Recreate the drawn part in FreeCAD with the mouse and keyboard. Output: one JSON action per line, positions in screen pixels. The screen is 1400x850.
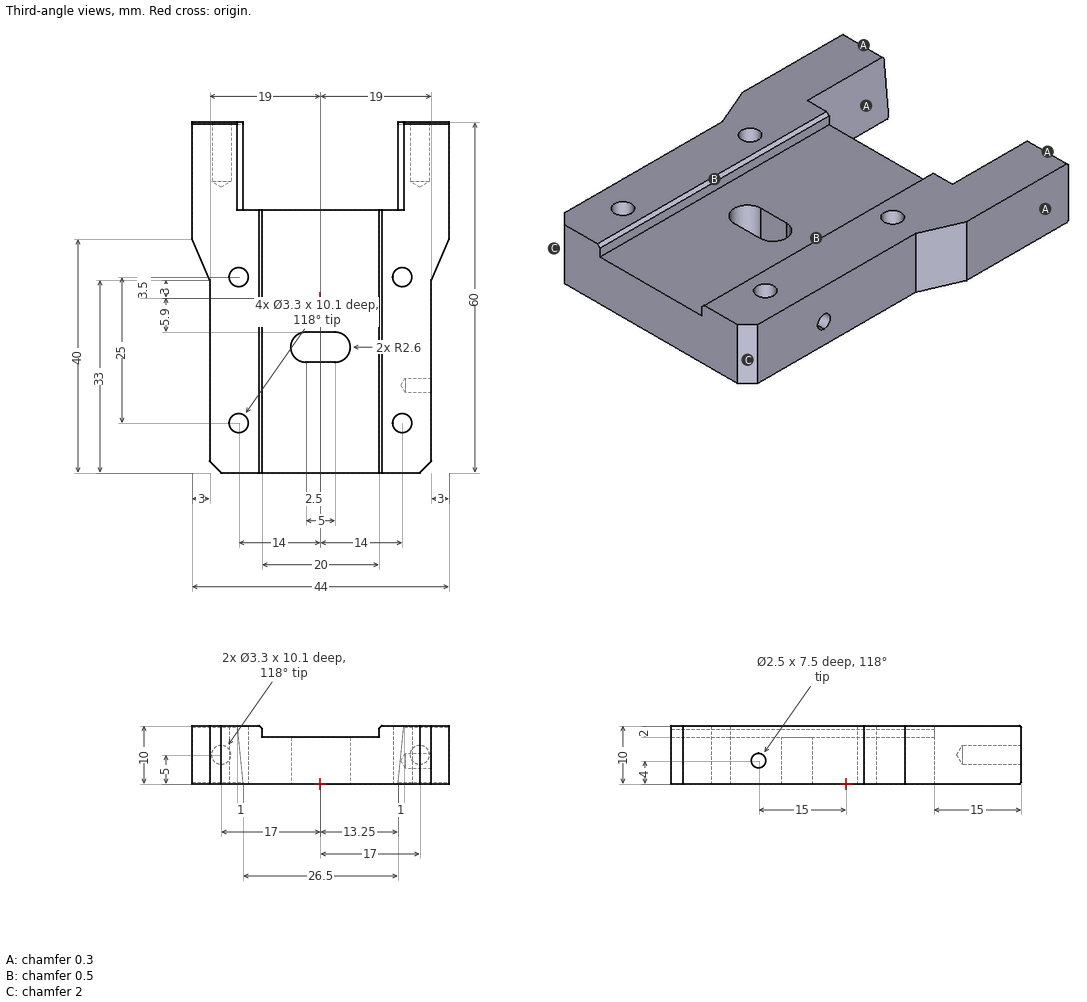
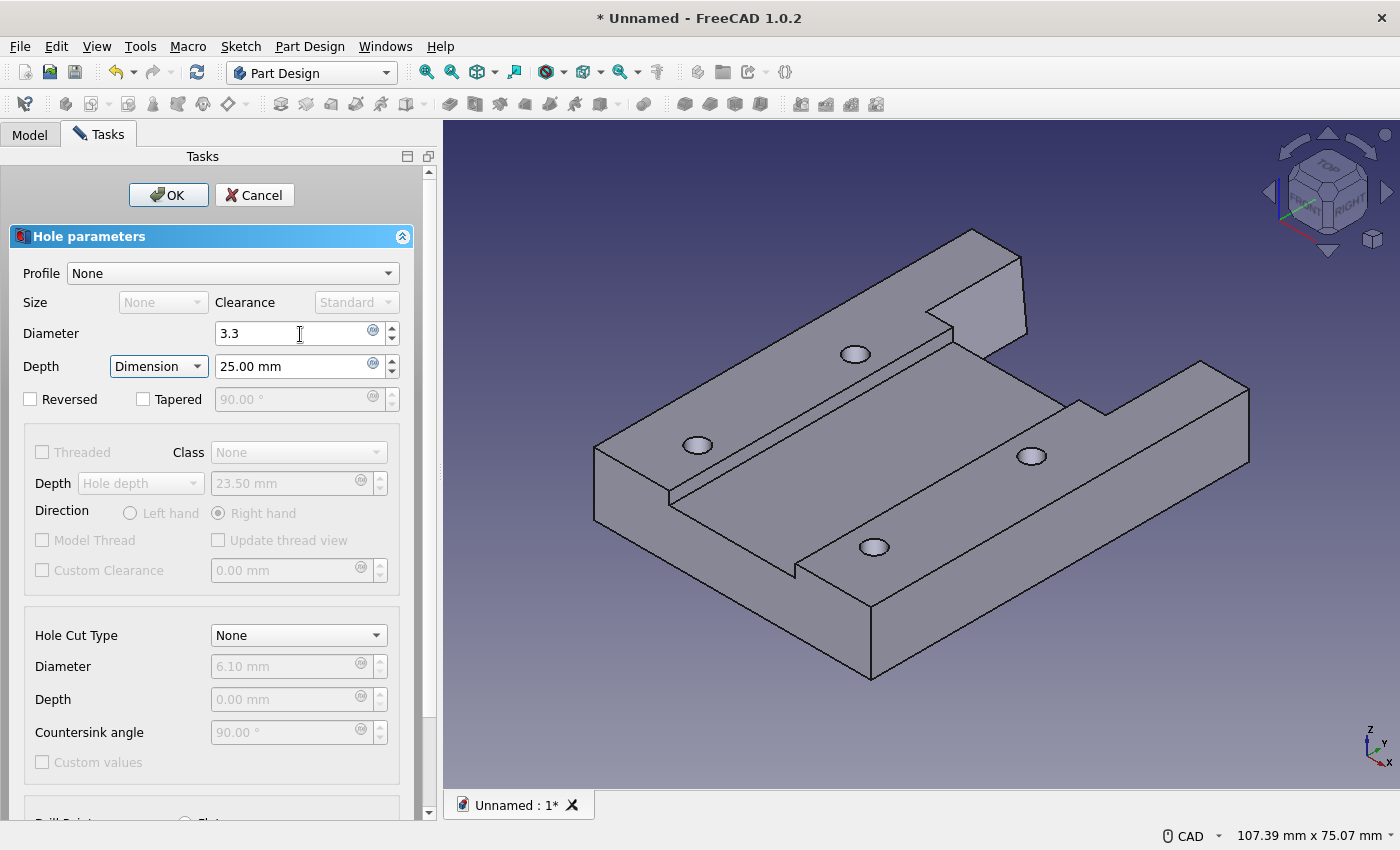
{"action": "triple_click", "coordinate": [300, 366]}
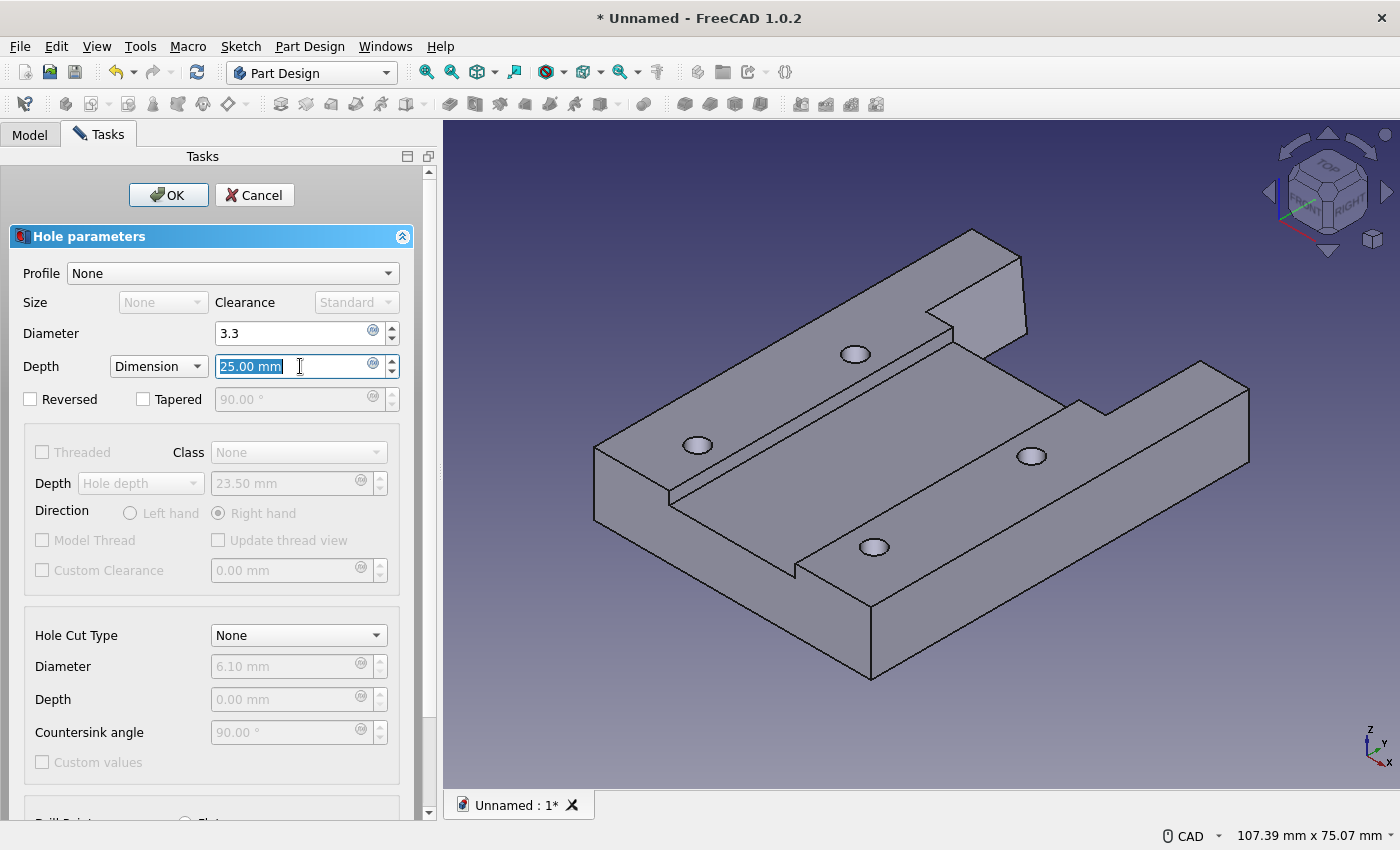
{"action": "type", "text": "10.1"}
{"action": "key", "text": "Tab"}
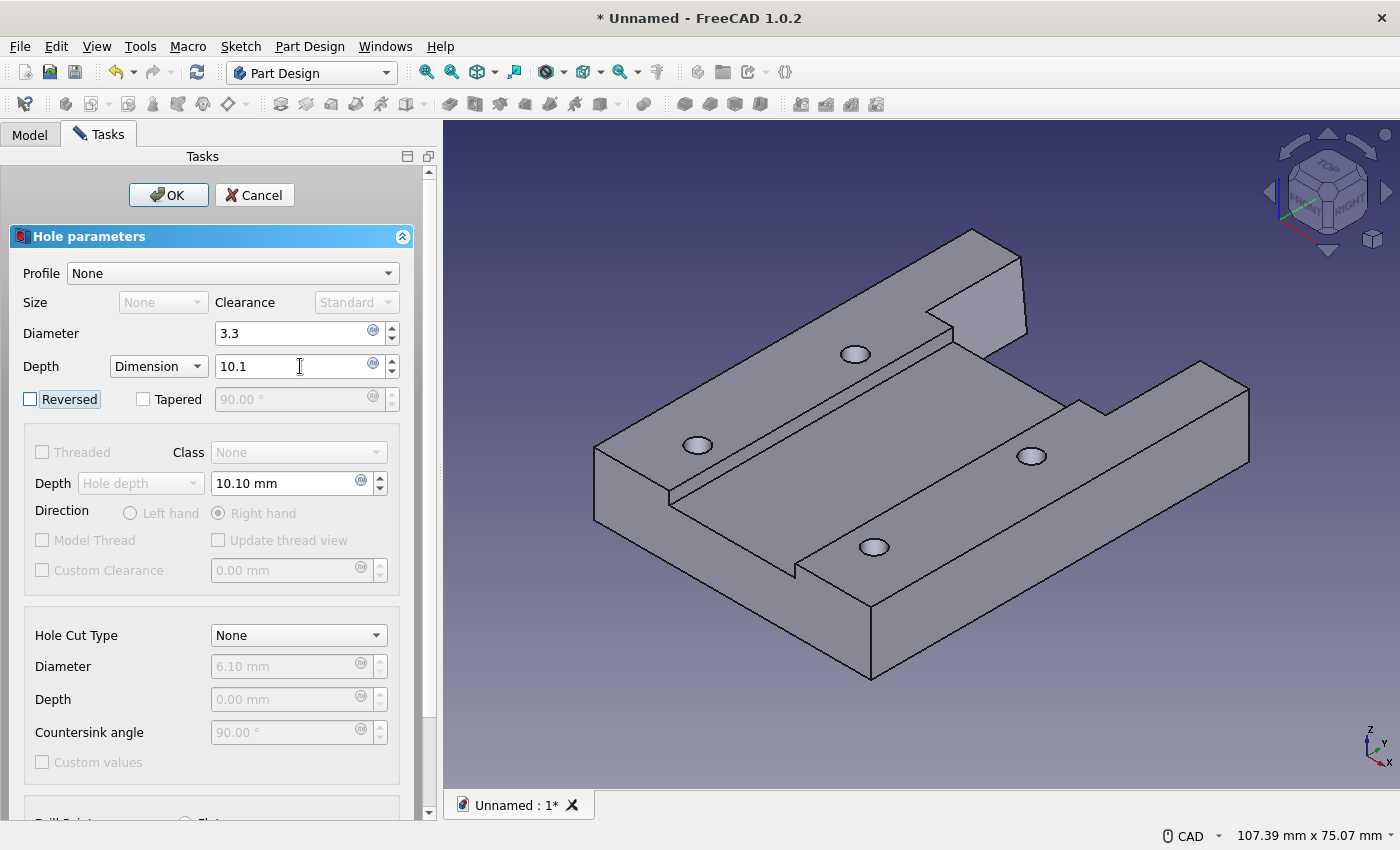
{"action": "left_click", "coordinate": [169, 195]}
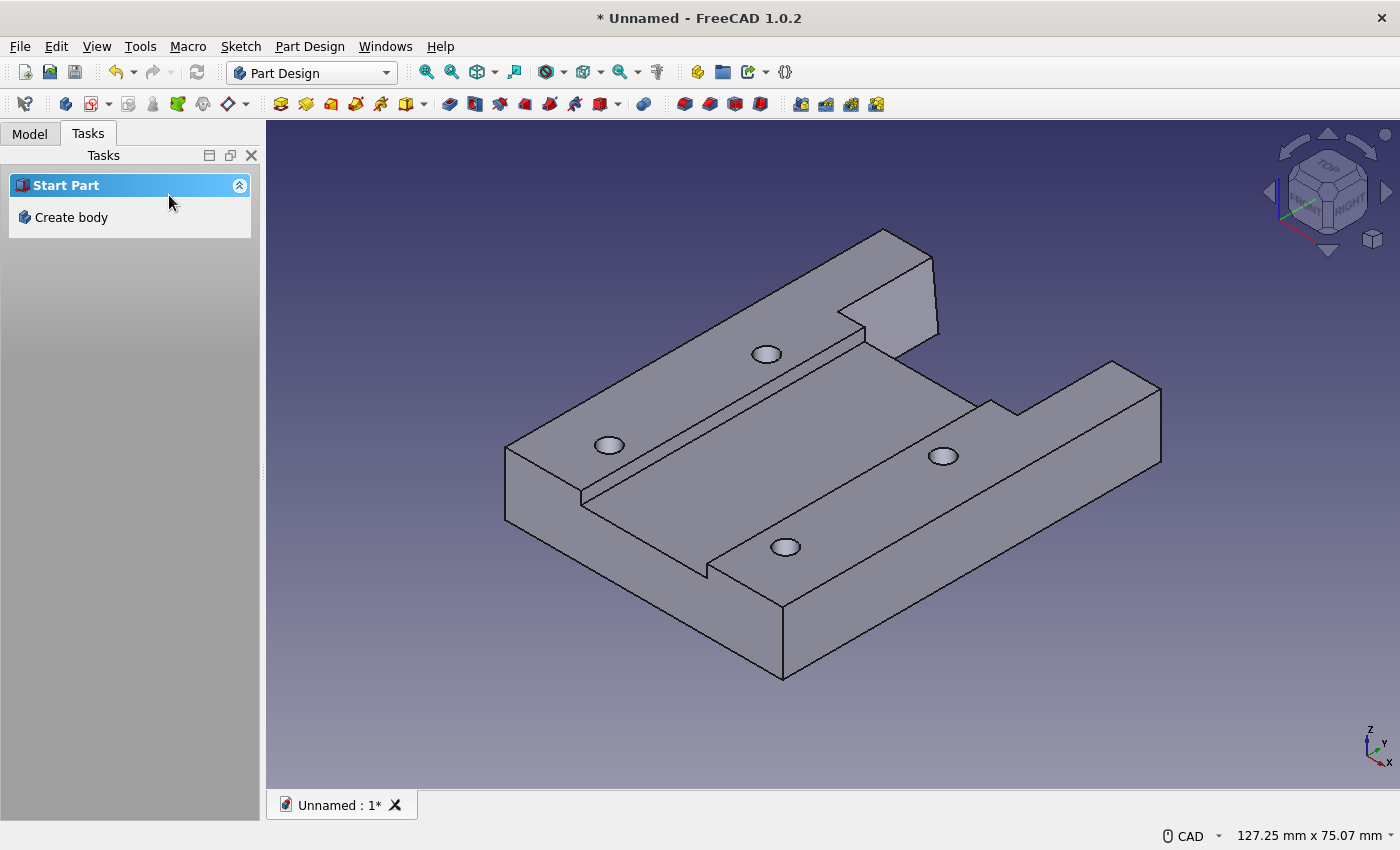
{"action": "left_click", "coordinate": [1080, 471]}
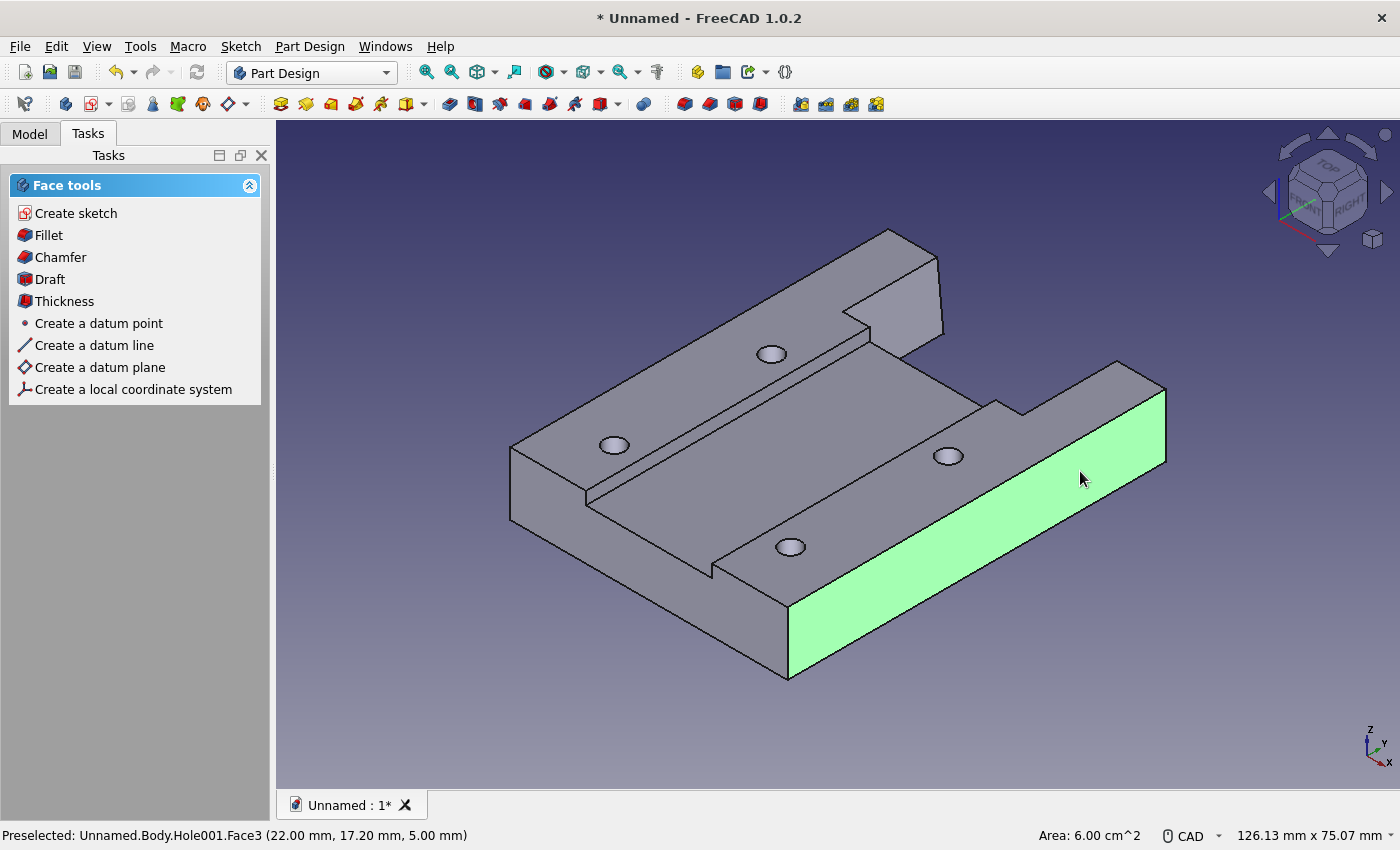
{"action": "left_click", "coordinate": [90, 104]}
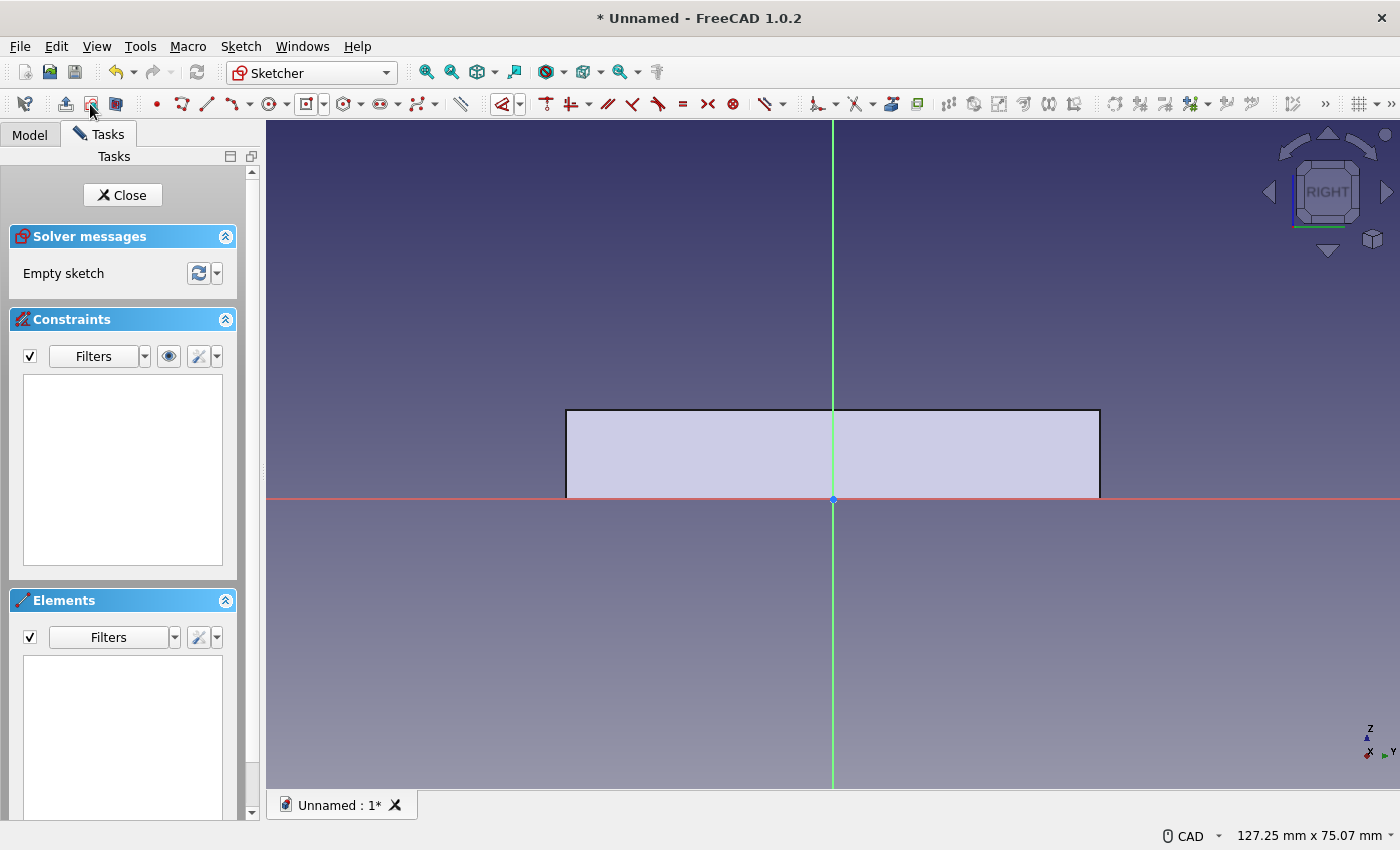
{"action": "scroll", "coordinate": [696, 464], "scroll_direction": "up", "scroll_amount": 15}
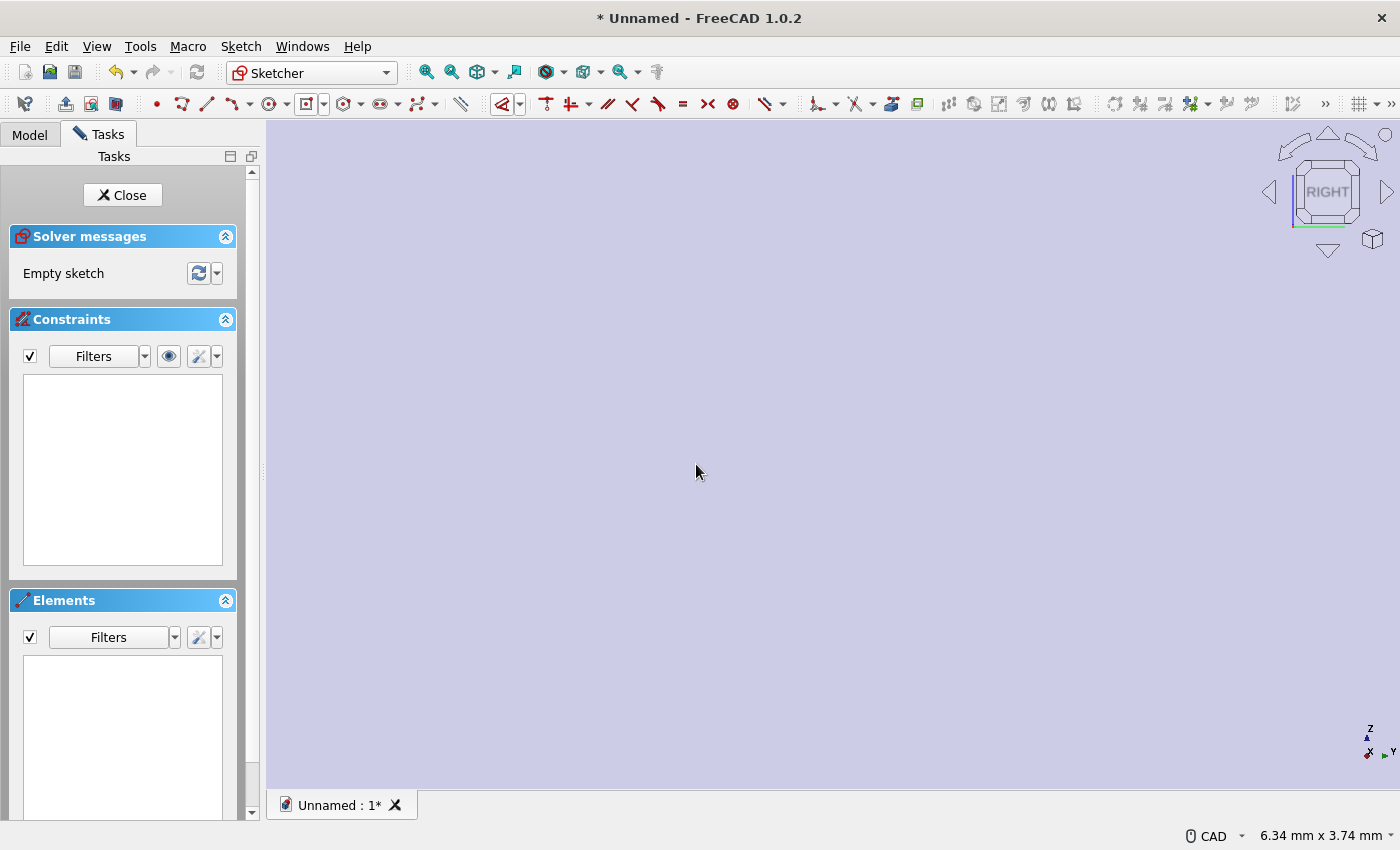
{"action": "key", "text": "g c"}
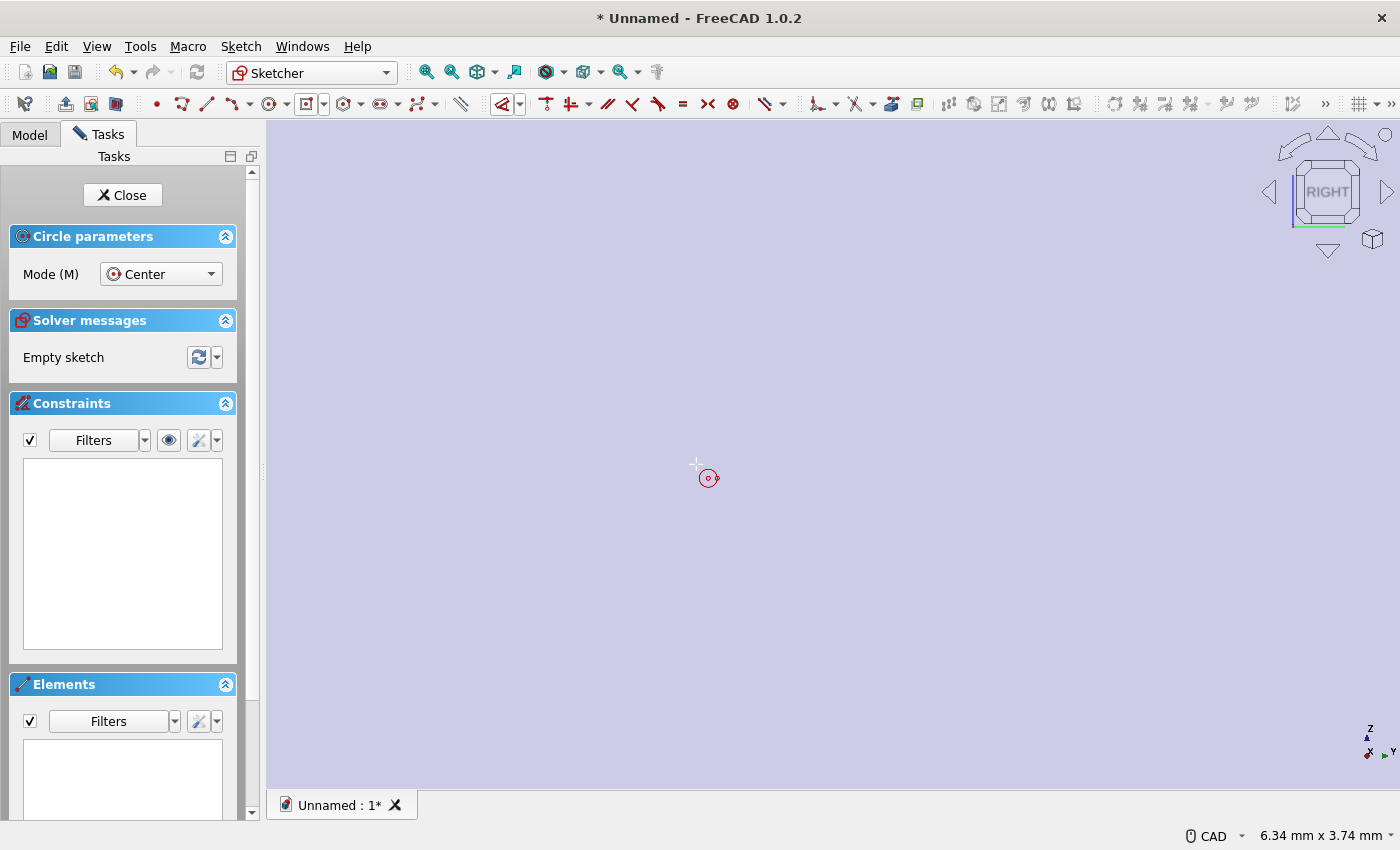
{"action": "left_click", "coordinate": [756, 442]}
{"action": "left_click", "coordinate": [914, 284]}
{"action": "key", "text": "Escape"}